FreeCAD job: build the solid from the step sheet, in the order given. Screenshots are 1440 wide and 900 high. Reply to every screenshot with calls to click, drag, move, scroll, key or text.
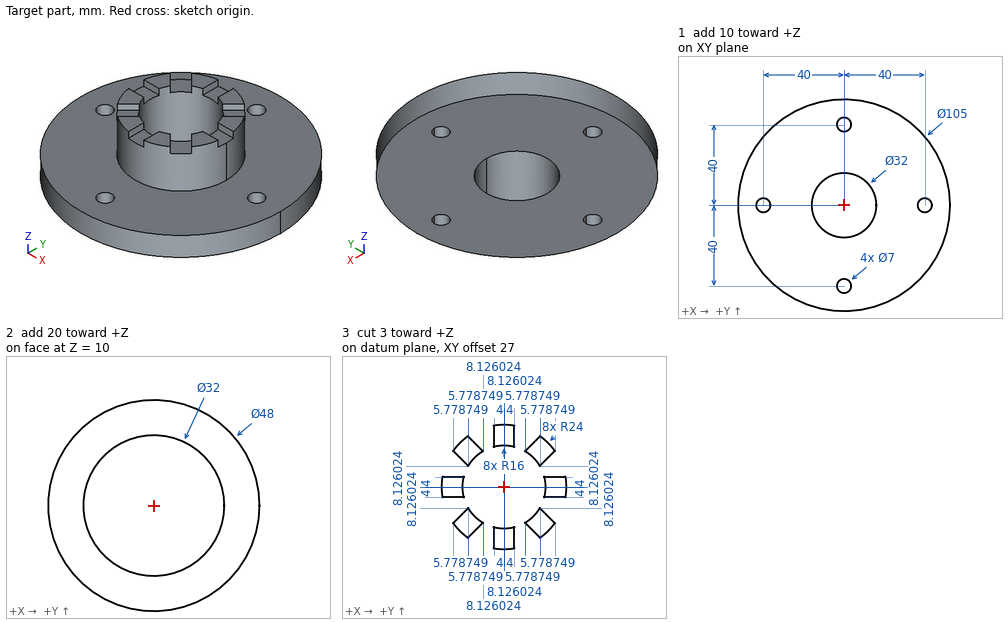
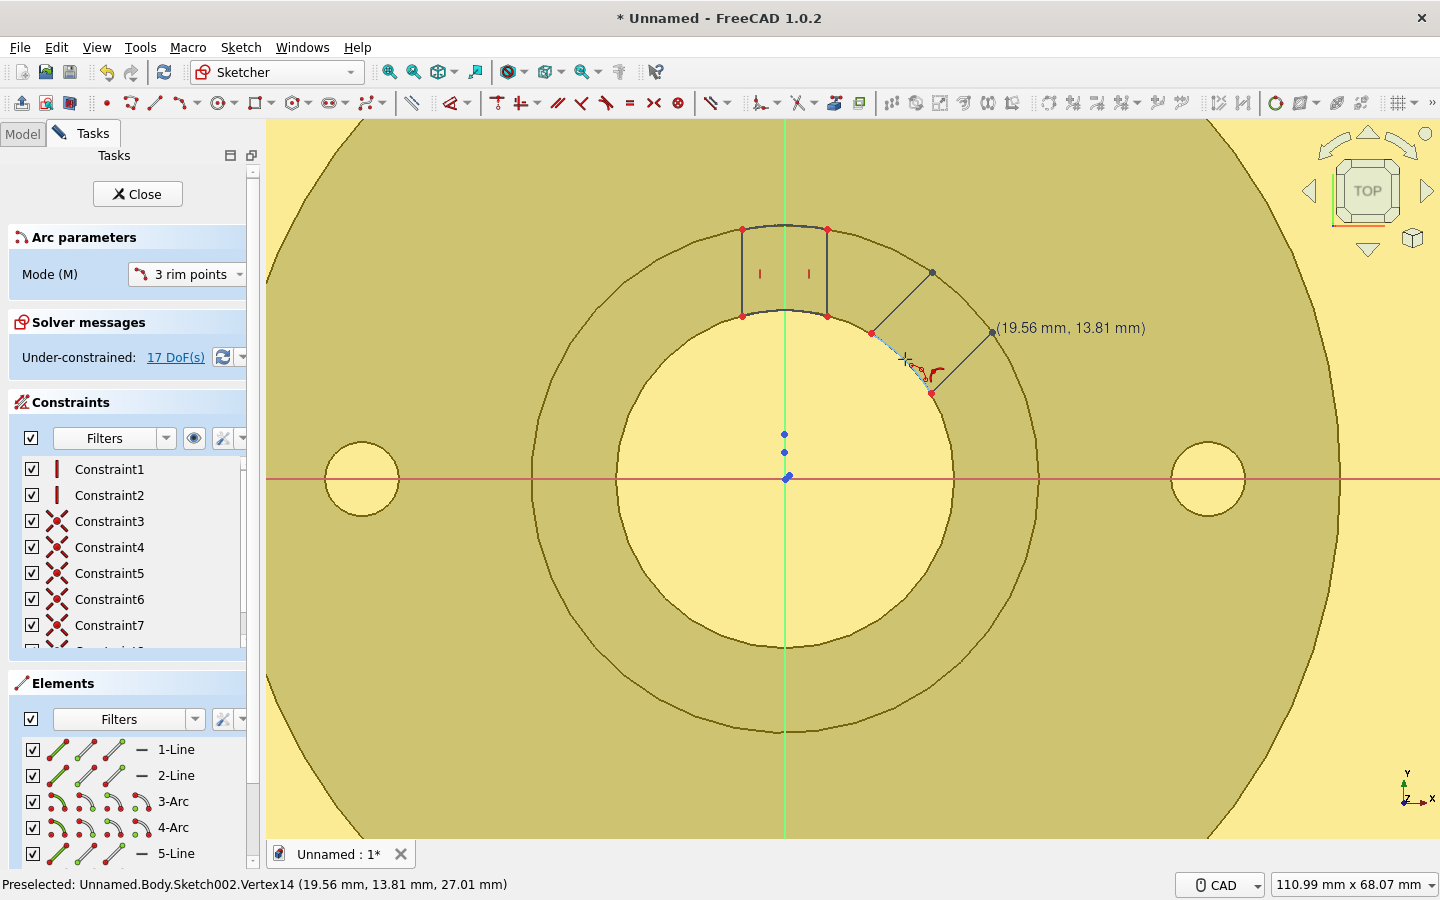
click(932, 273)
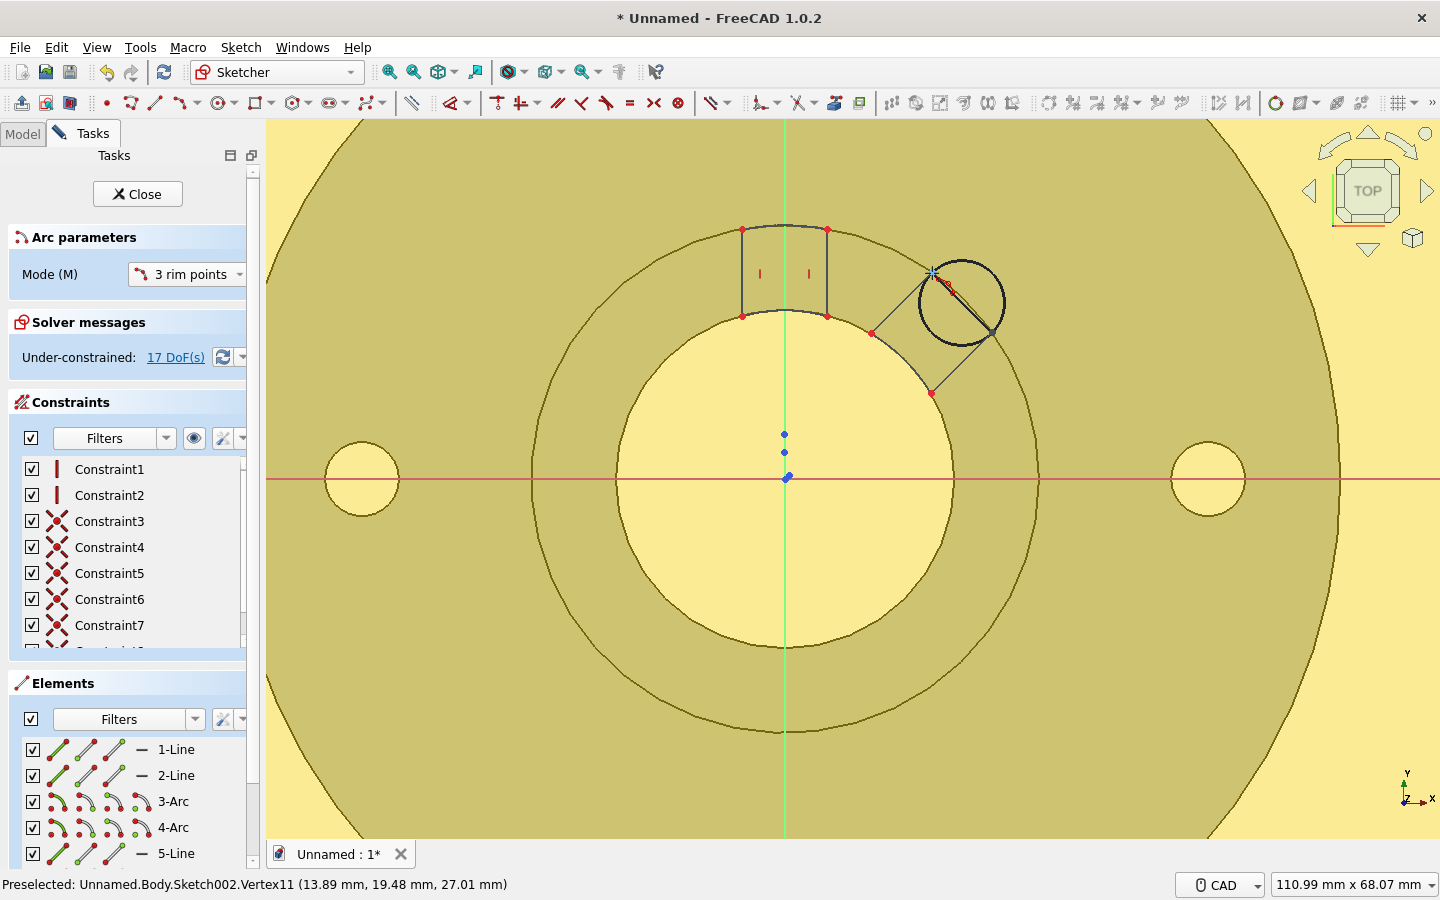
scroll(965, 300, up, 8)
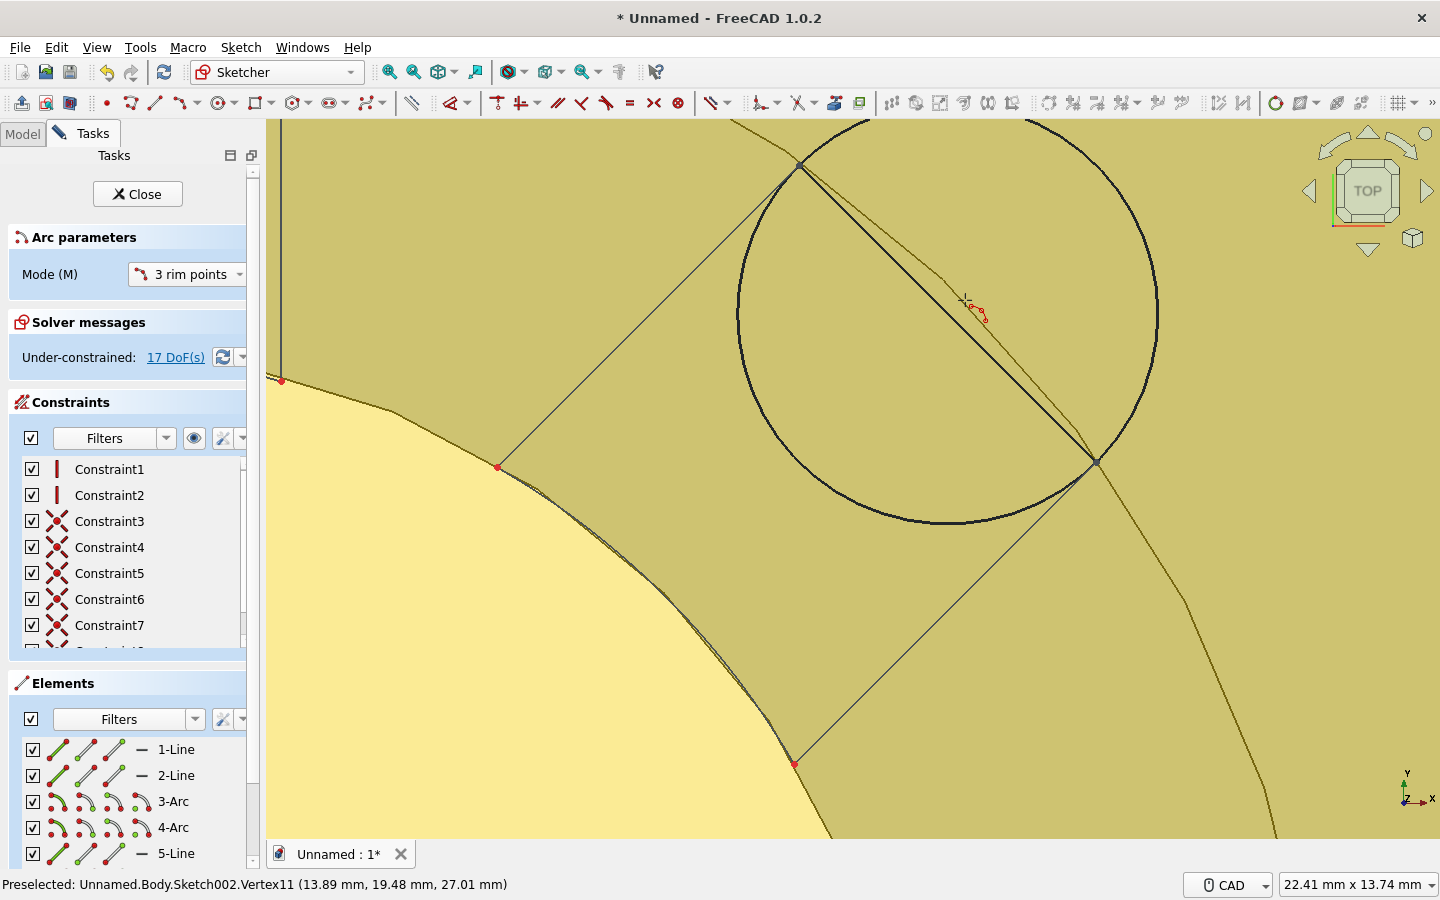
click(961, 297)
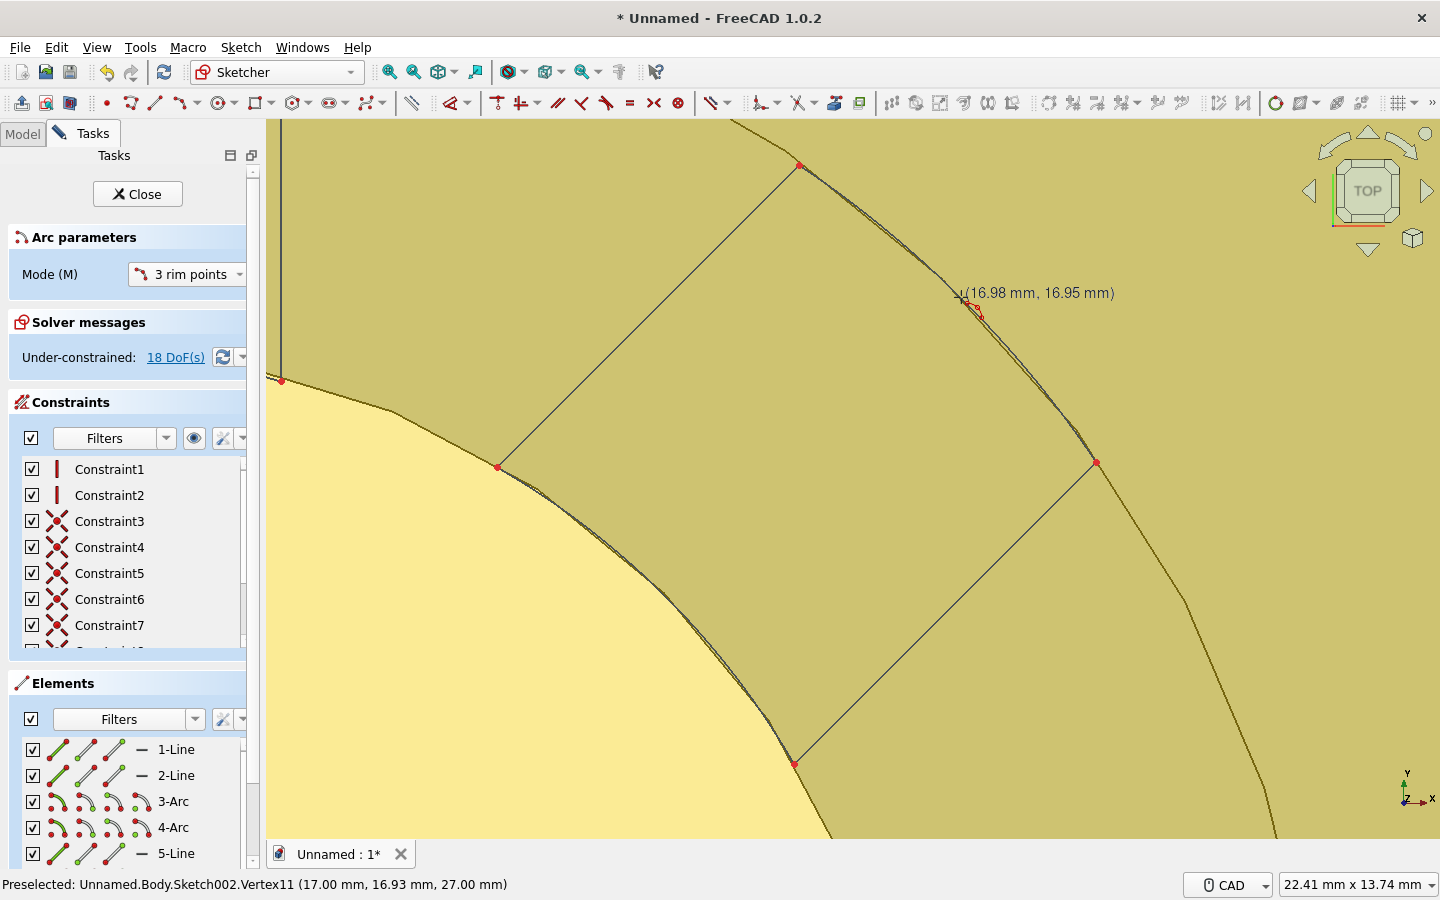
click(156, 104)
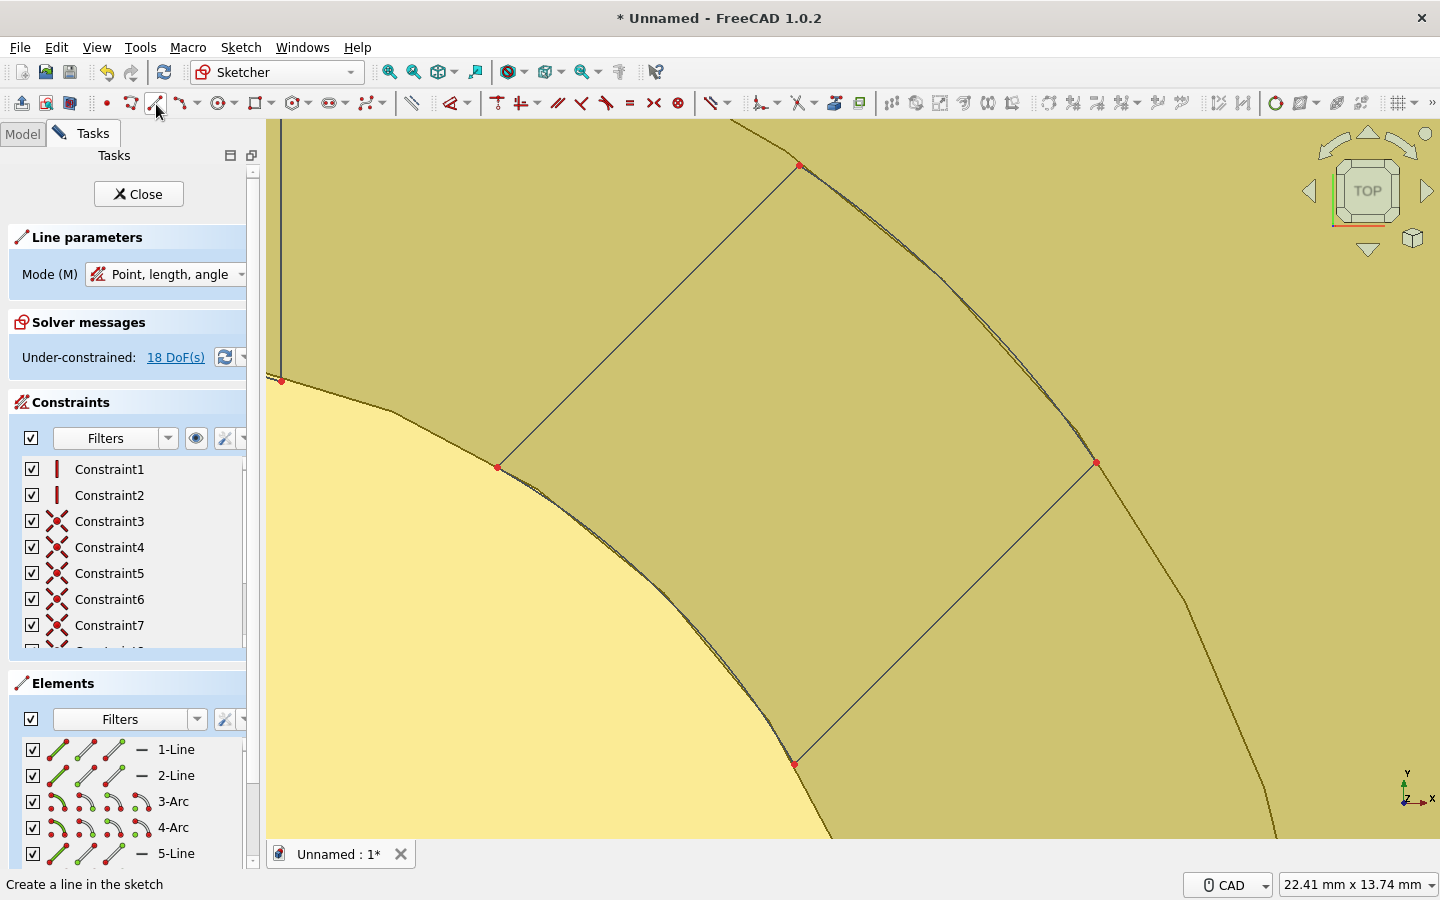
scroll(965, 300, down, 8)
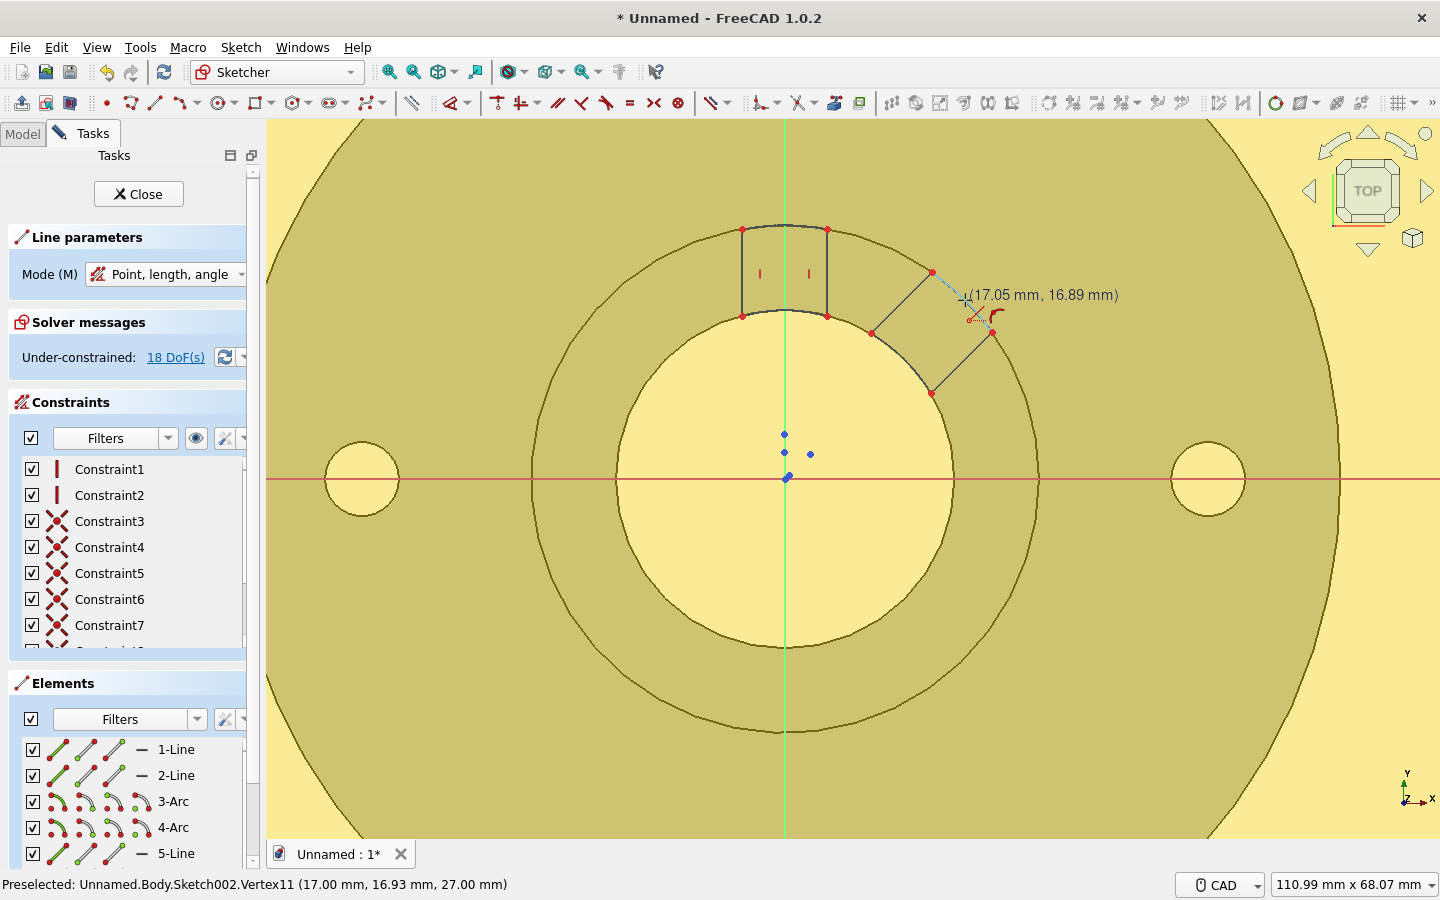
click(1035, 437)
click(949, 437)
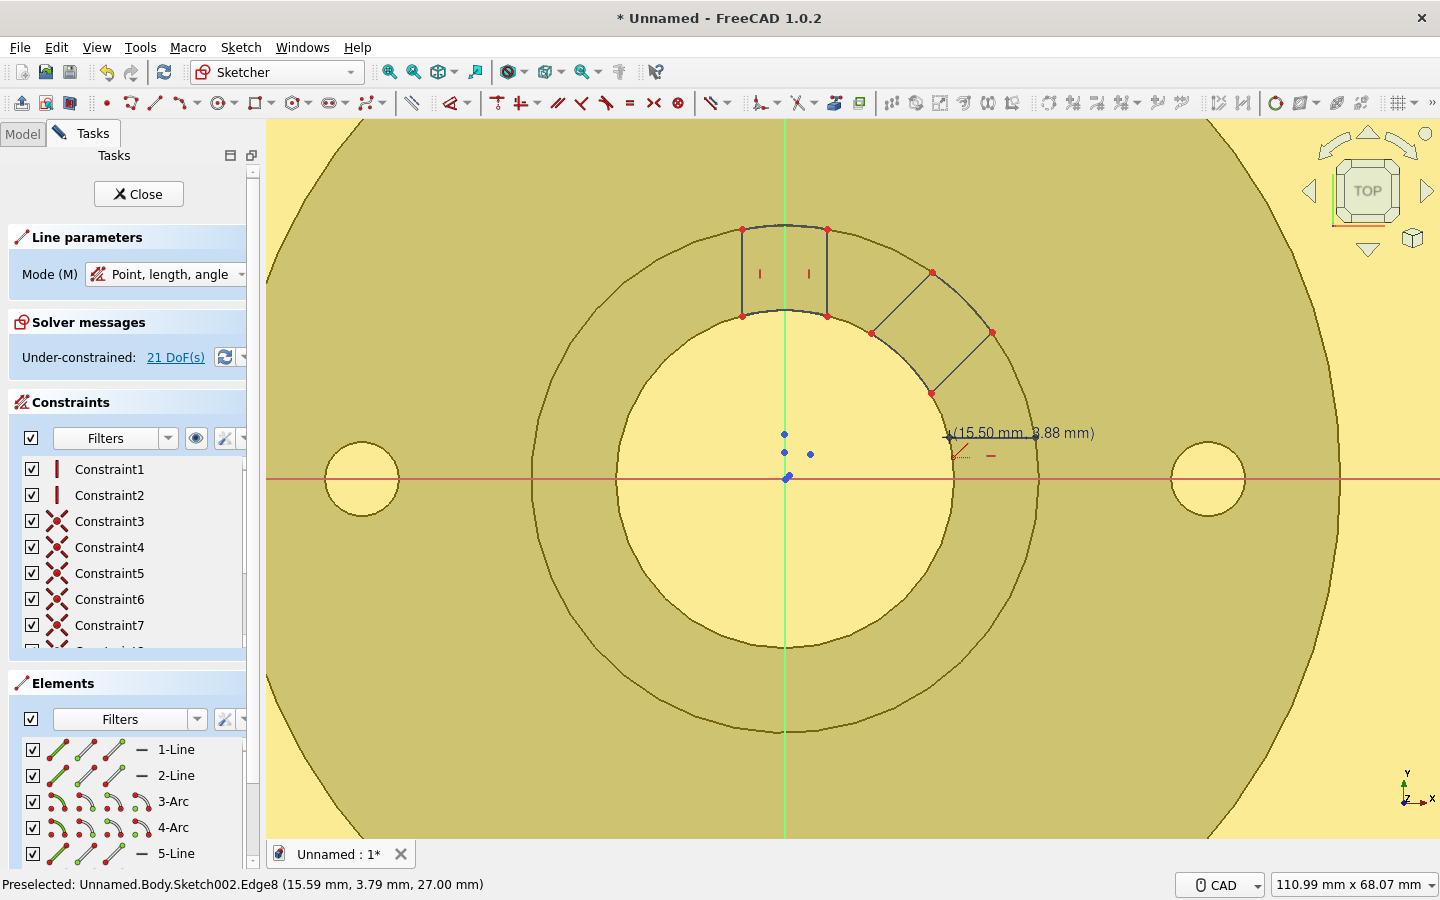
click(949, 521)
click(1035, 521)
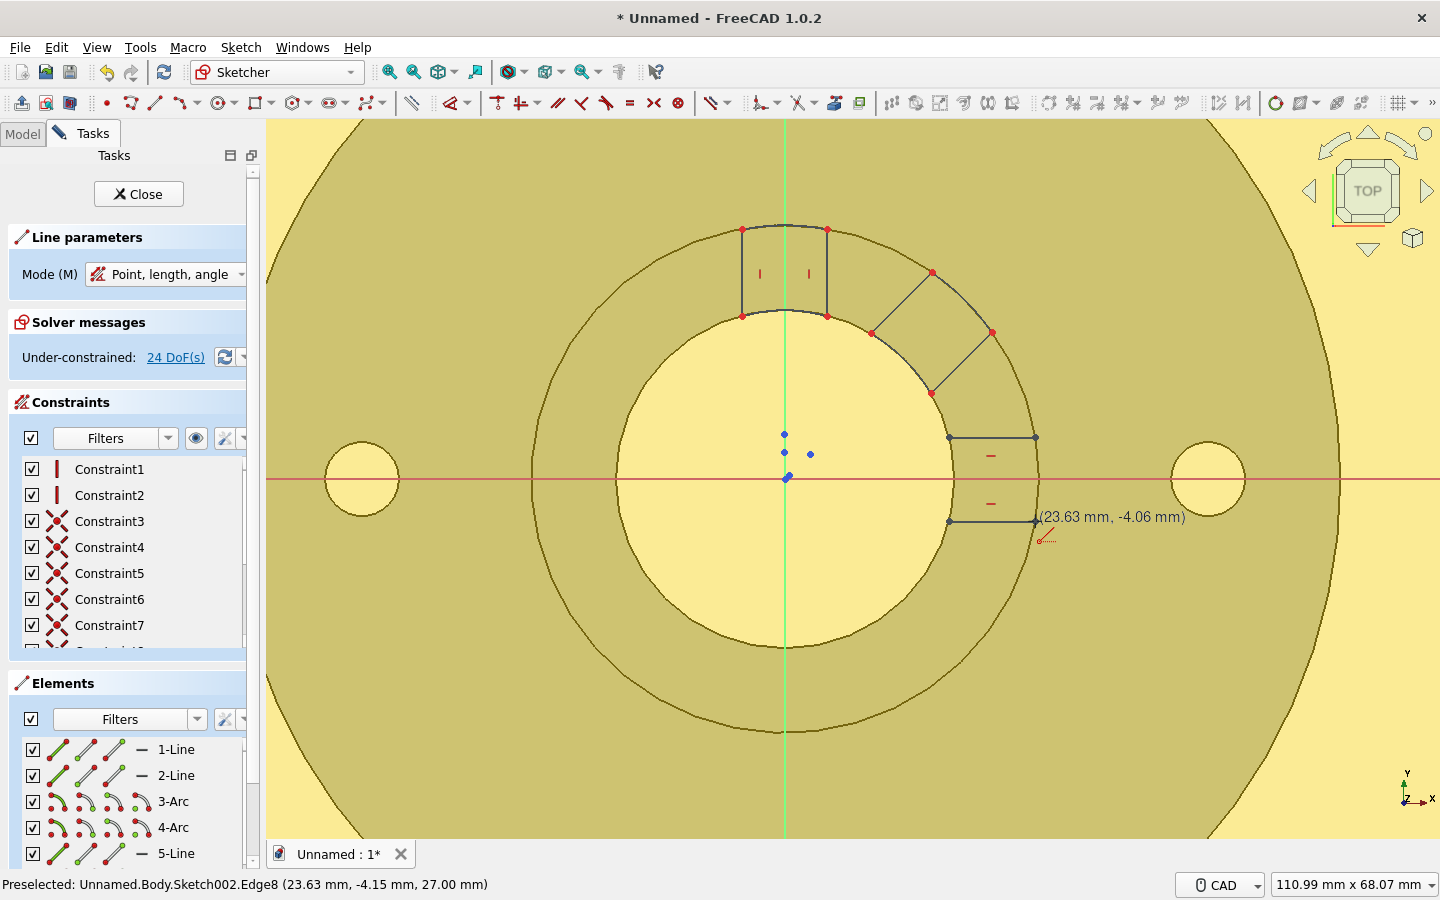
click(180, 104)